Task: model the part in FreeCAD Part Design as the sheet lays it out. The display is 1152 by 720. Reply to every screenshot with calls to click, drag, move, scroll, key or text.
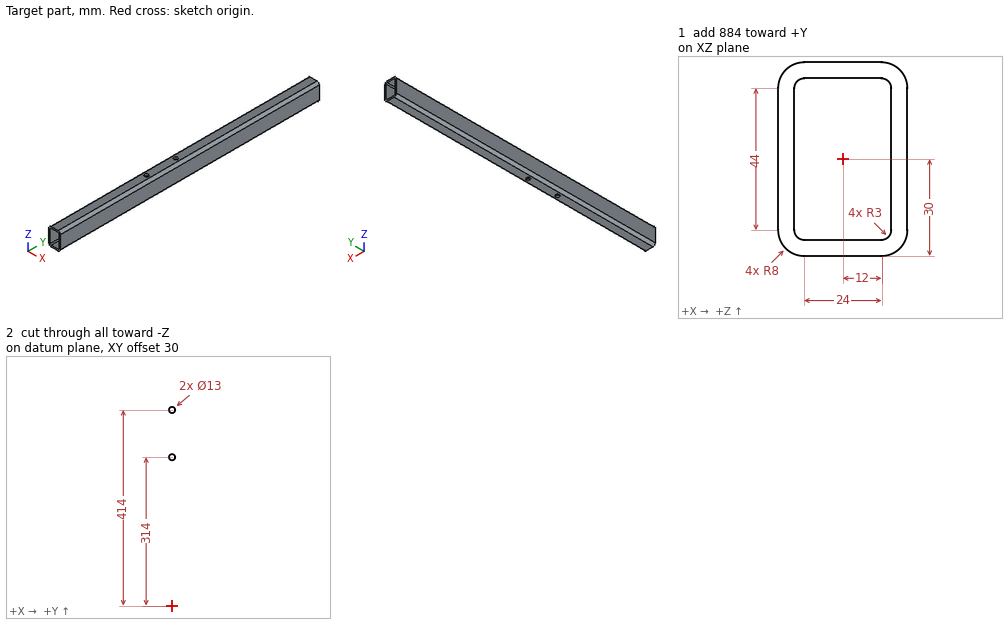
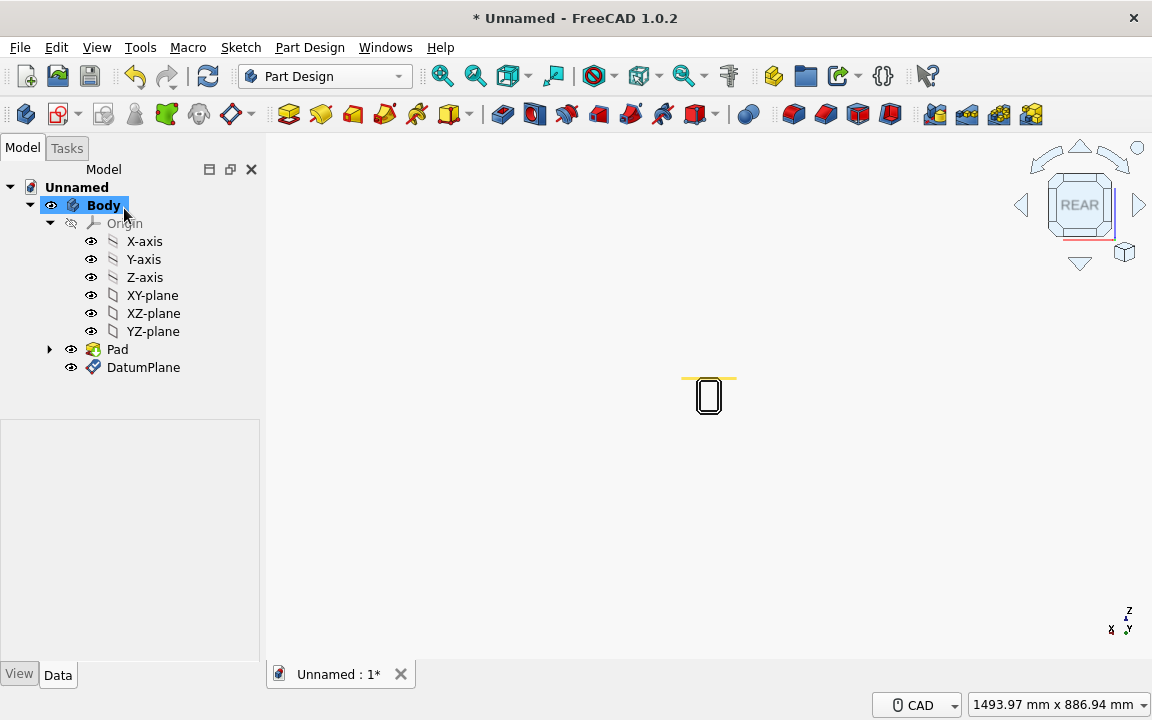
click(116, 367)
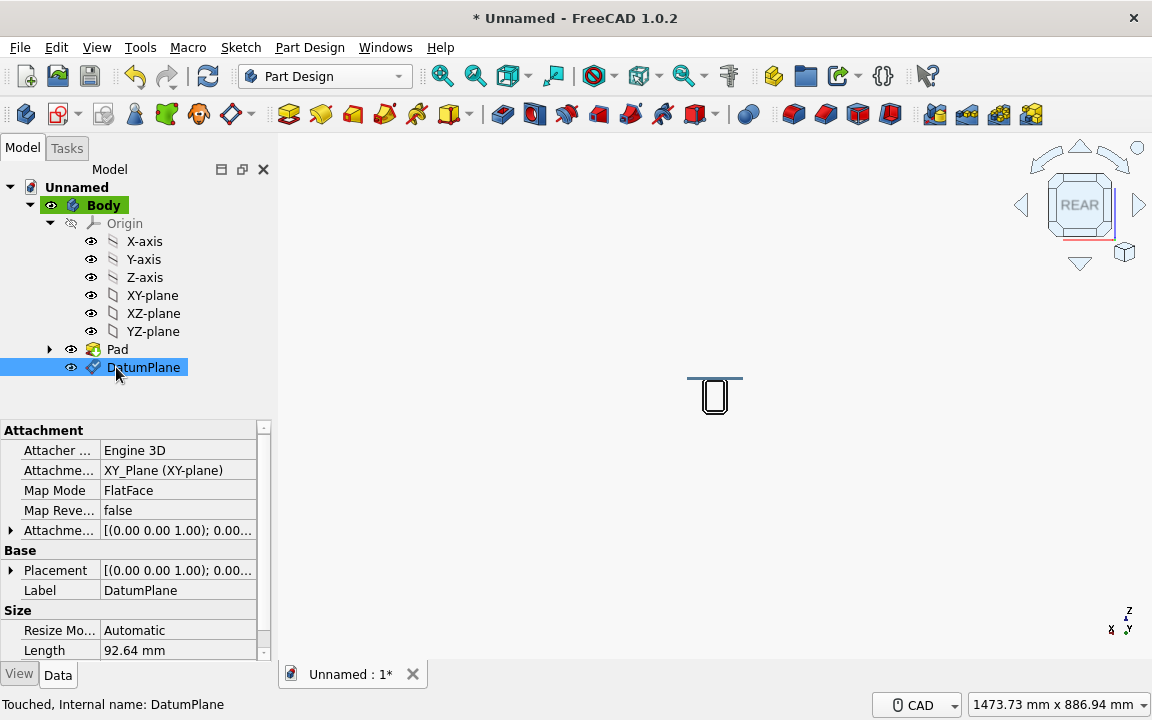
click(58, 114)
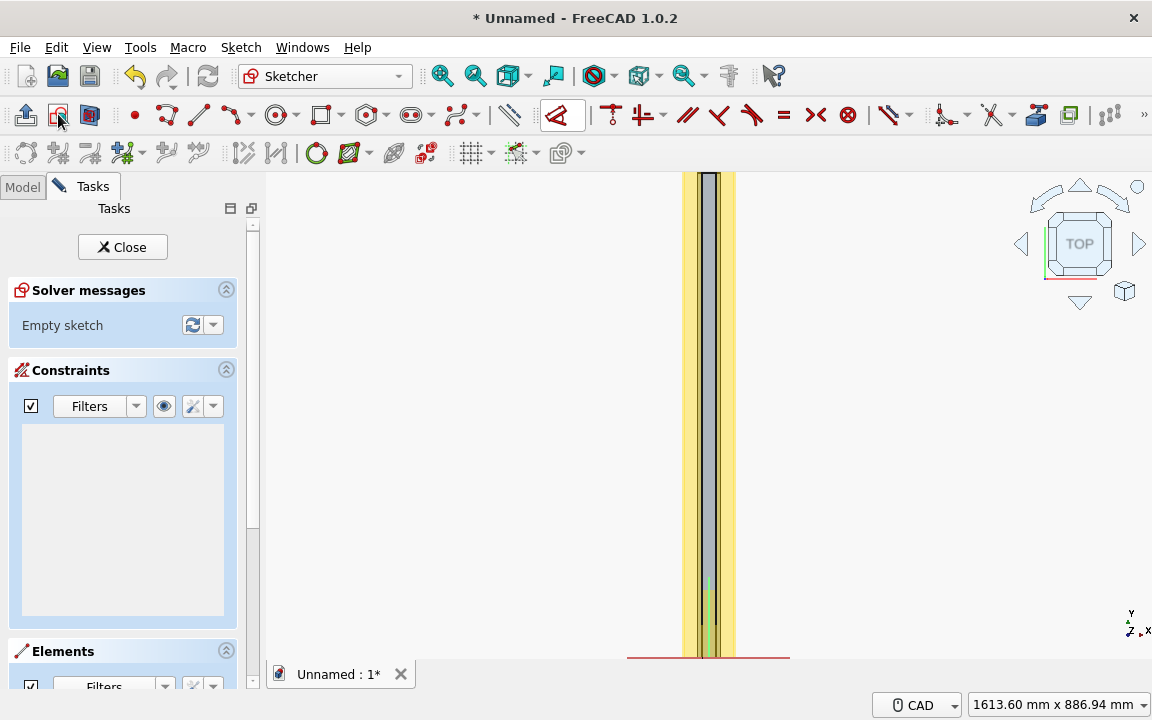
scroll(726, 469, up, 8)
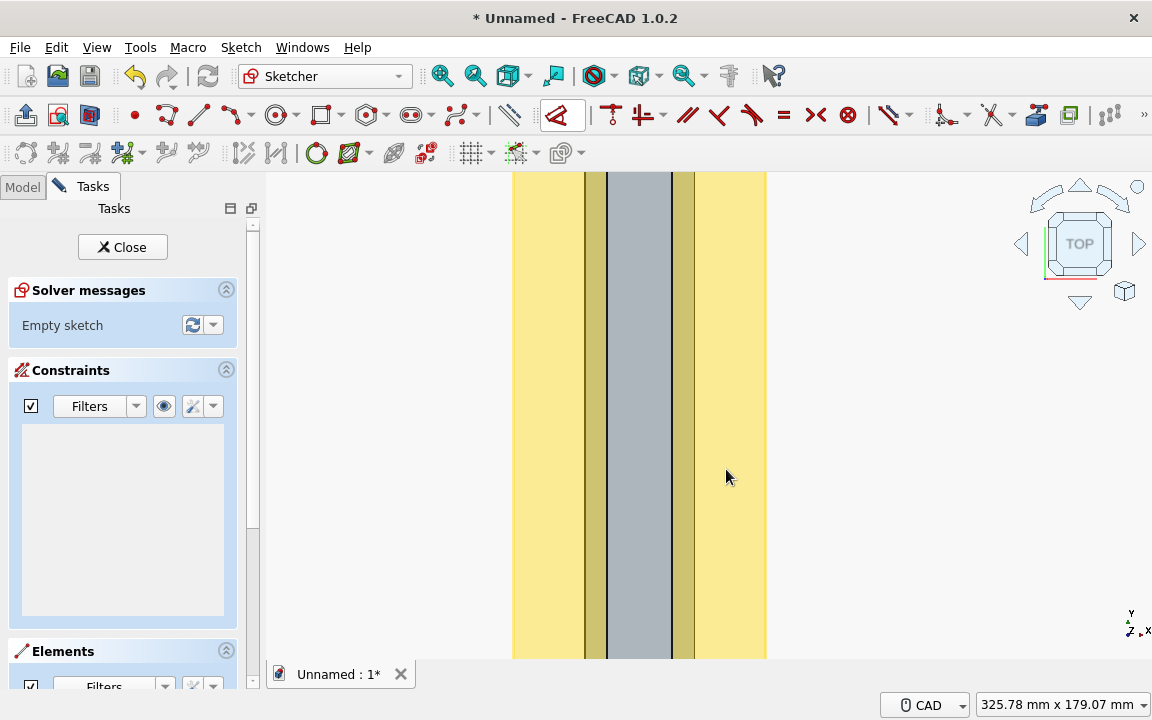
key(g)
key(c)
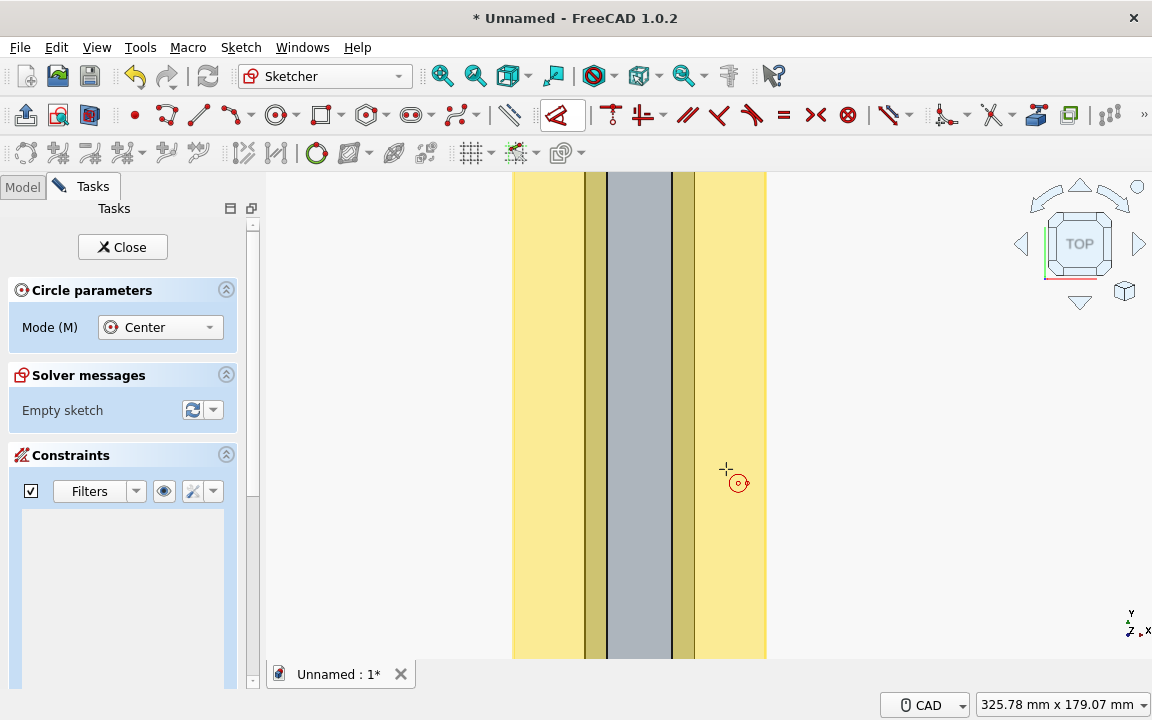
scroll(640, 278, up, 2)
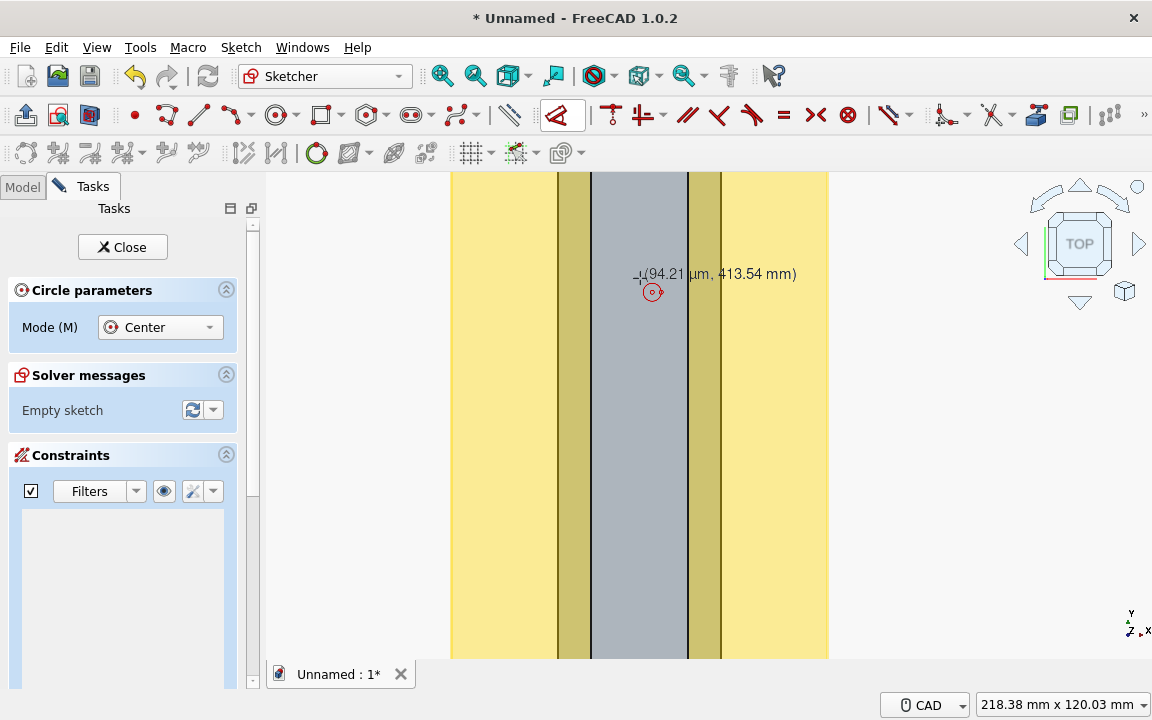
click(639, 278)
move(658, 259)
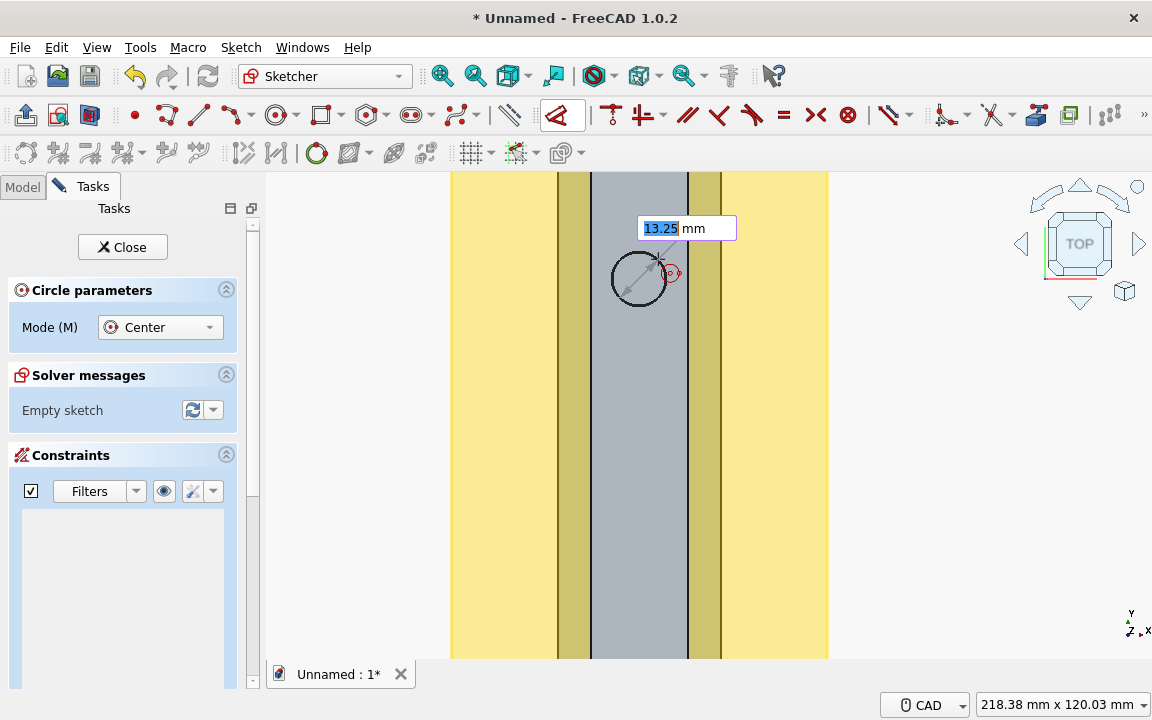
text(13)
key(Return)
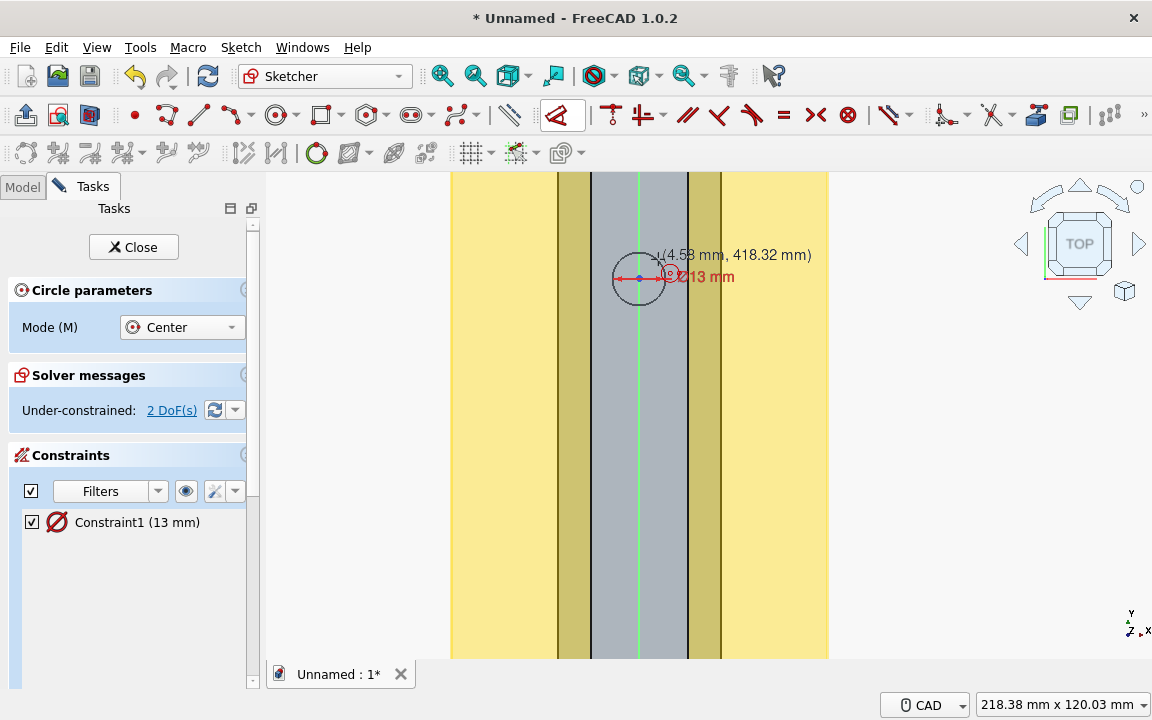
scroll(643, 284, down, 2)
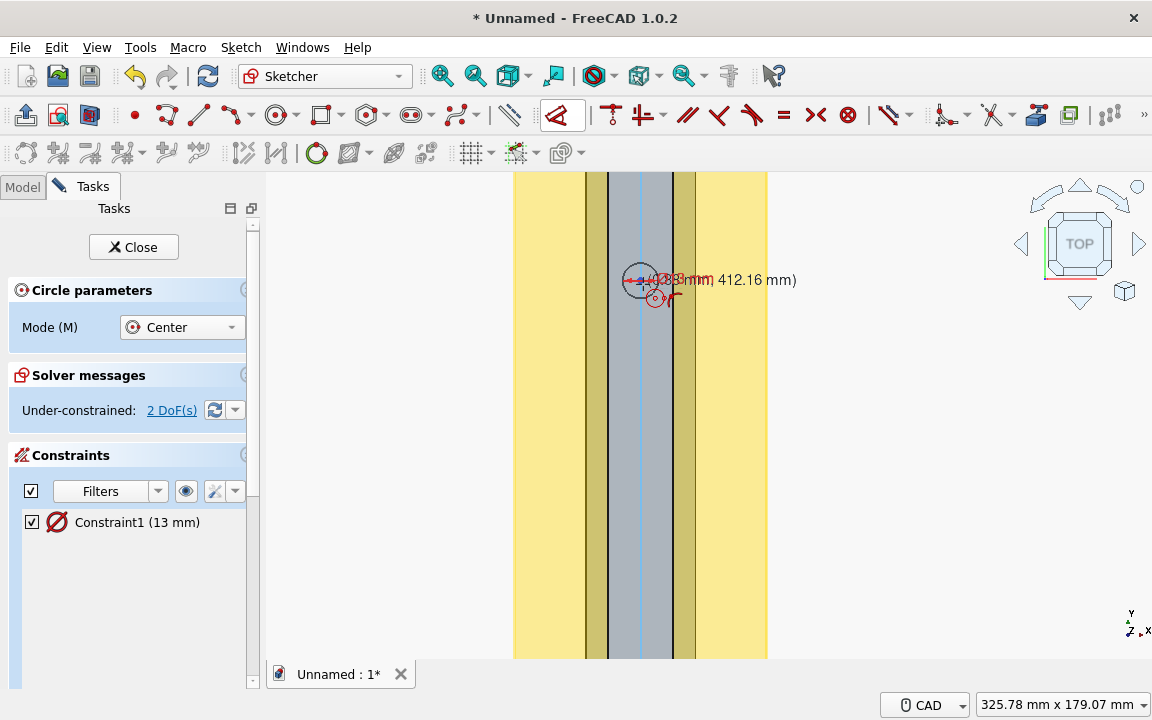
scroll(641, 552, up, 2)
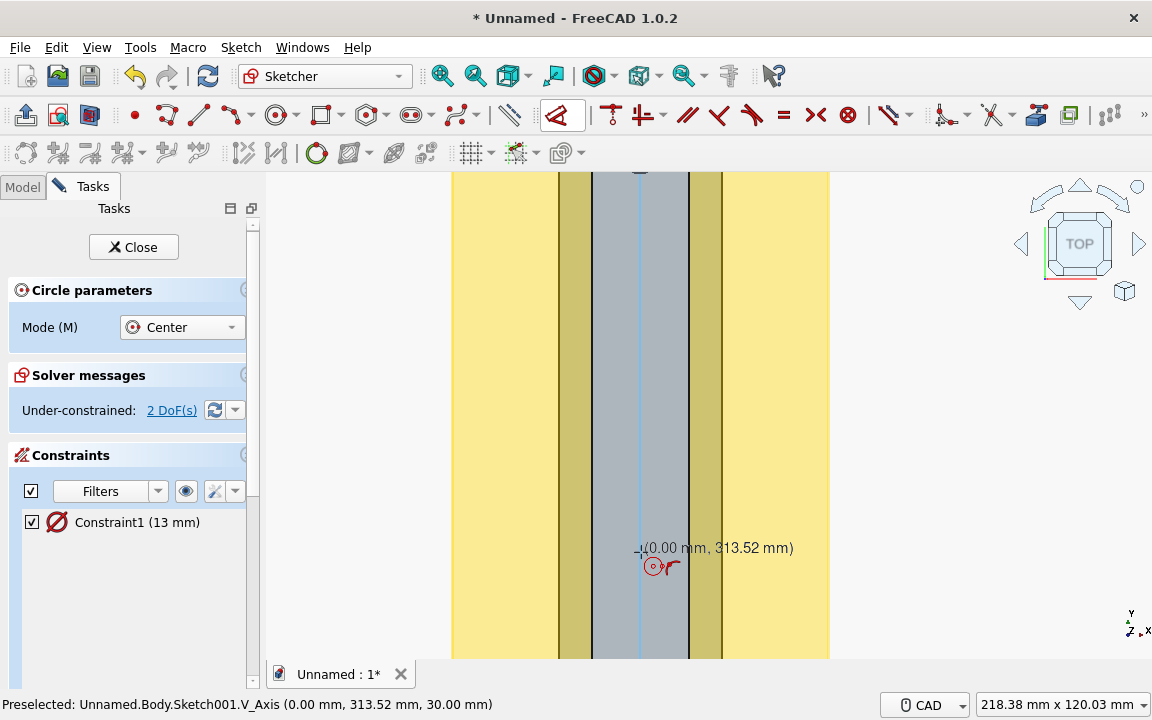
click(640, 551)
move(659, 533)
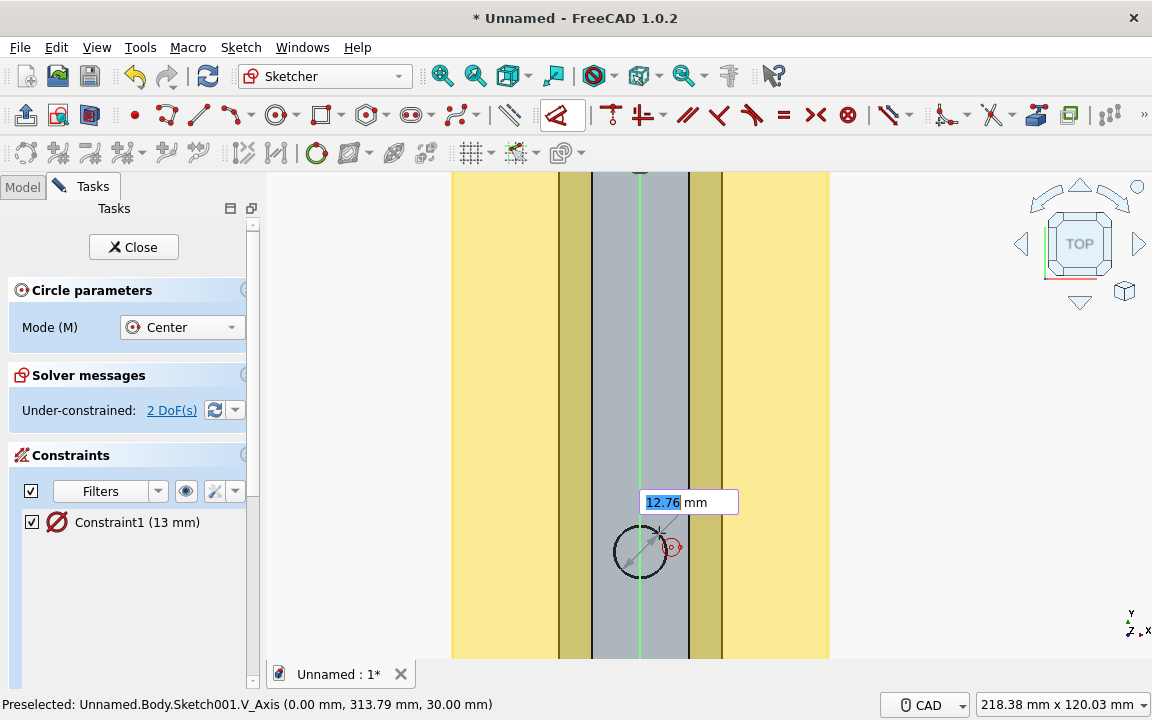
text(13)
key(Return)
key(Escape)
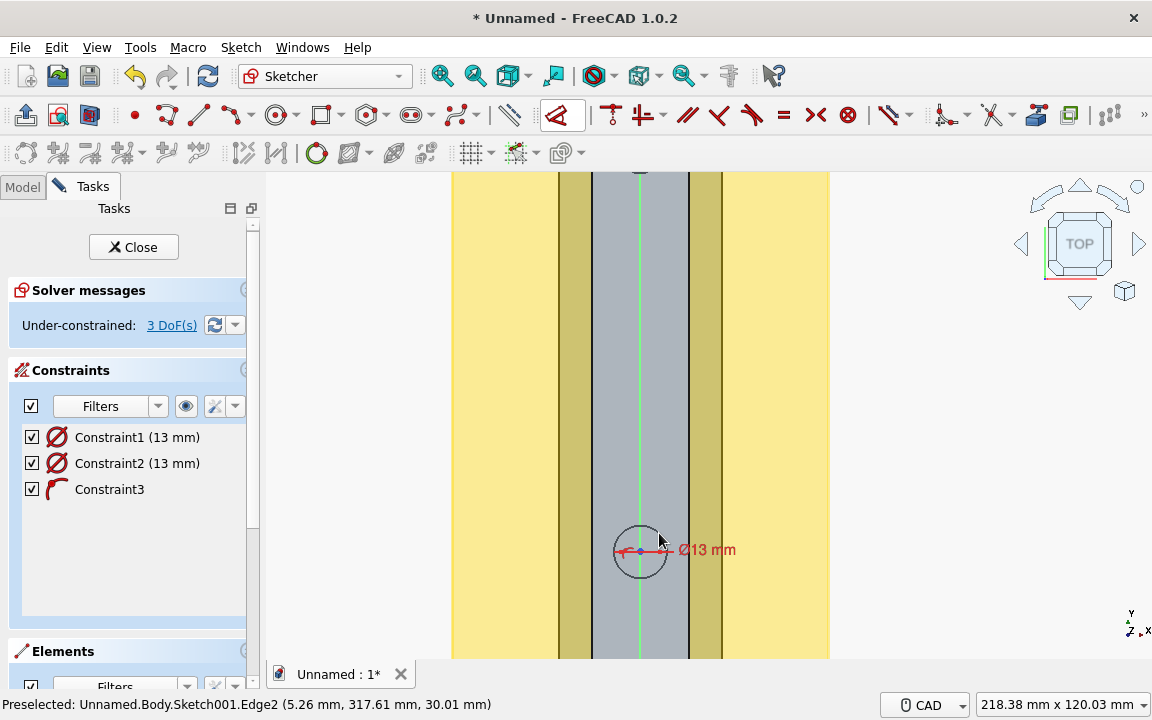
scroll(641, 552, down, 2)